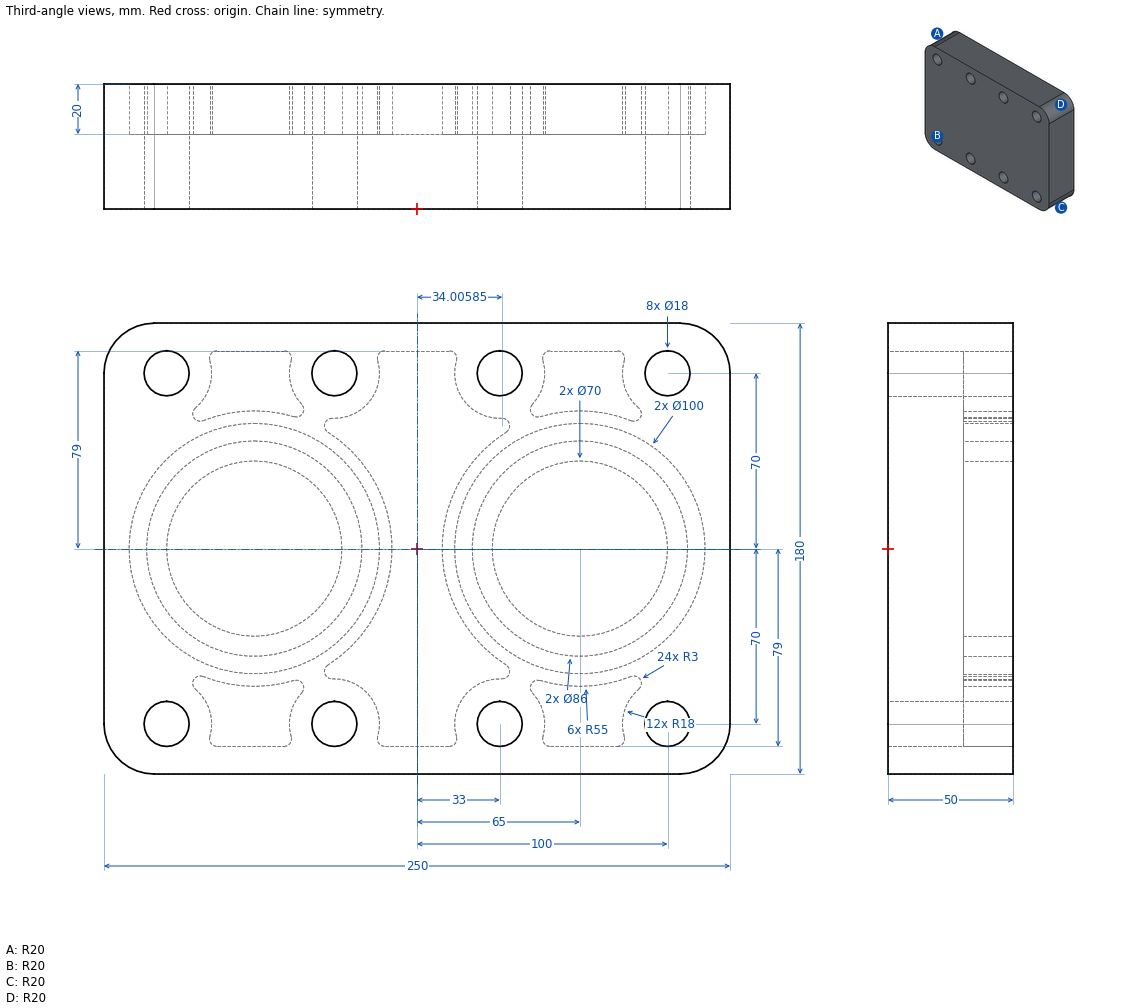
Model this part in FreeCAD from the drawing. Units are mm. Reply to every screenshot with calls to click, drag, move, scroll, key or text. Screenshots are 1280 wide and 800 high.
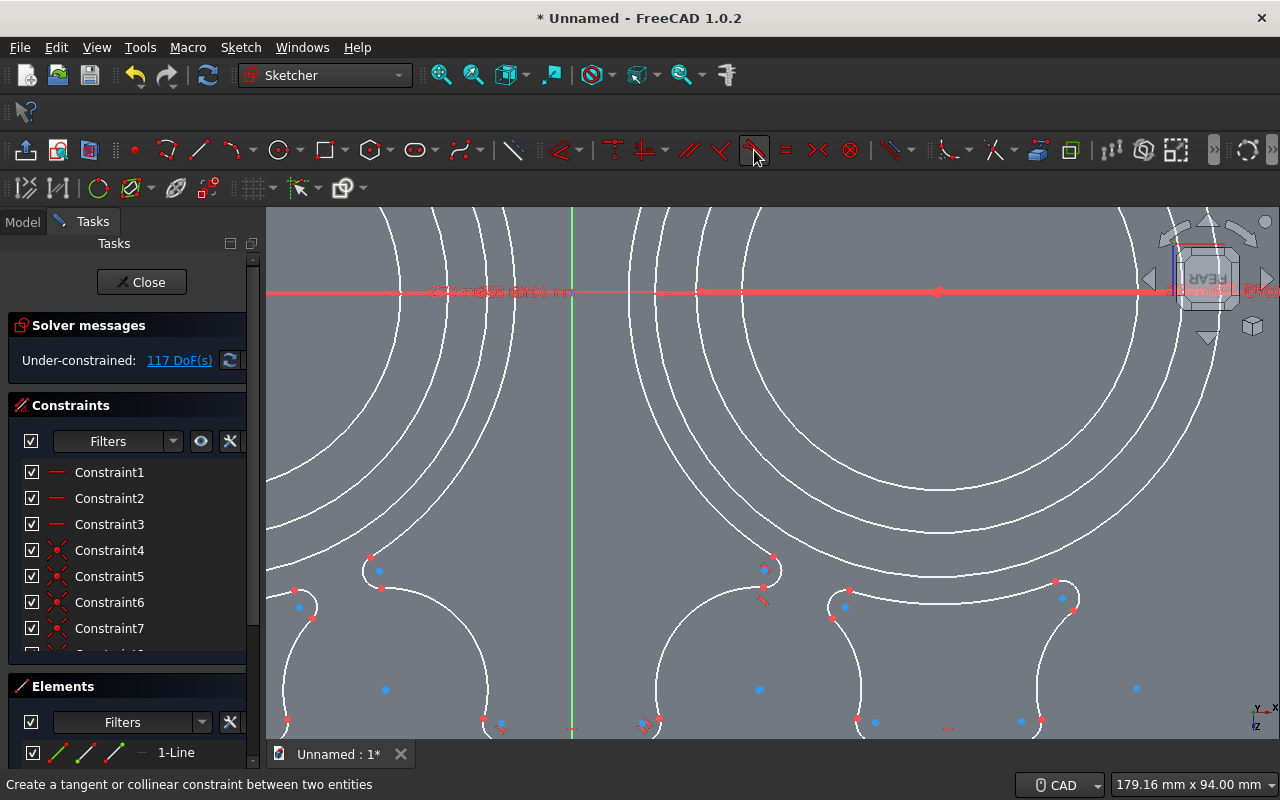
click(654, 416)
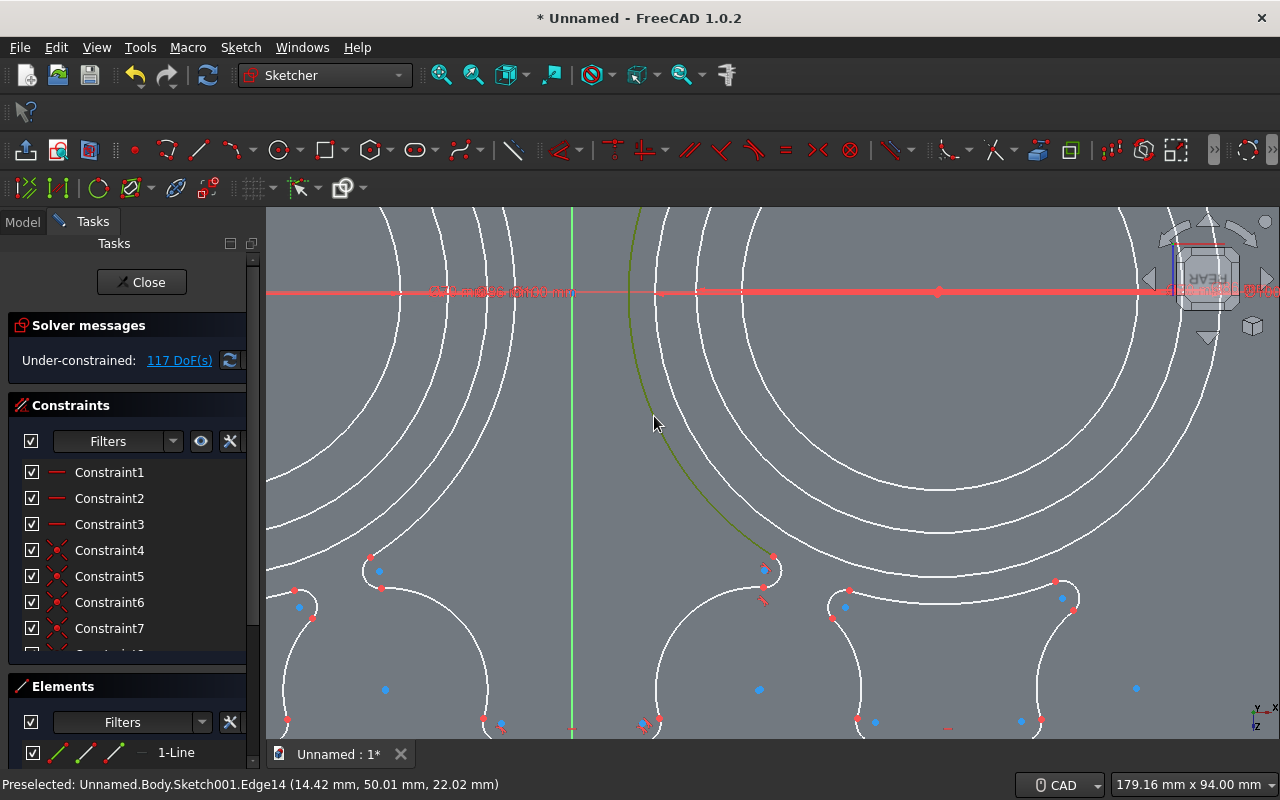
scroll(781, 578, down, 5)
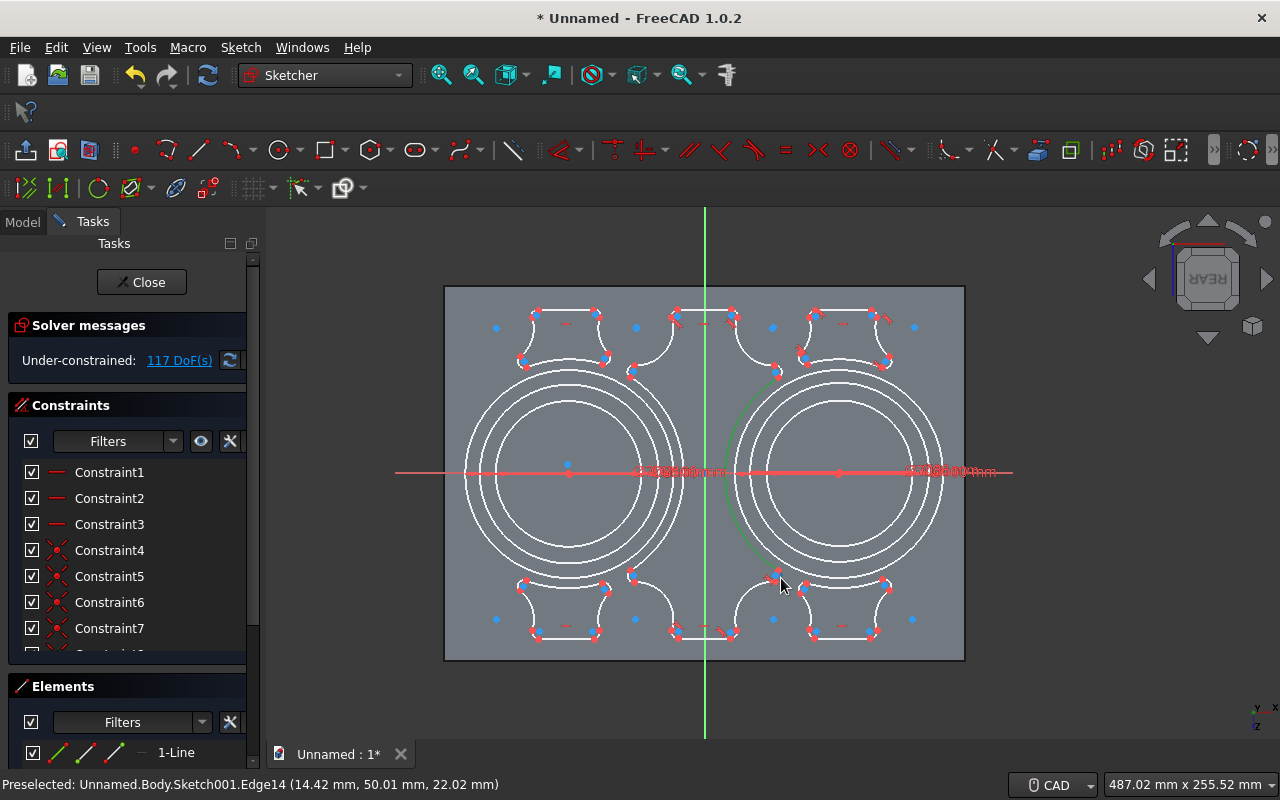
scroll(782, 374, up, 5)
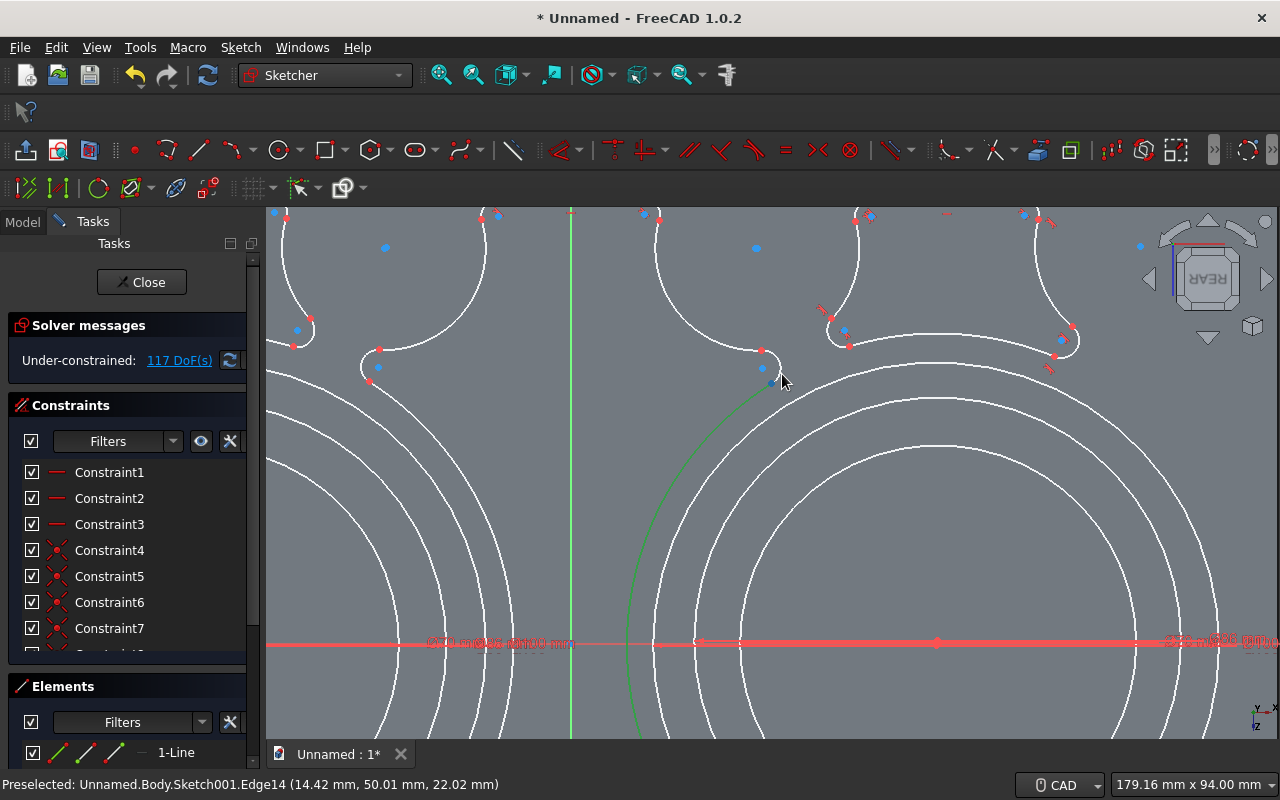
click(780, 373)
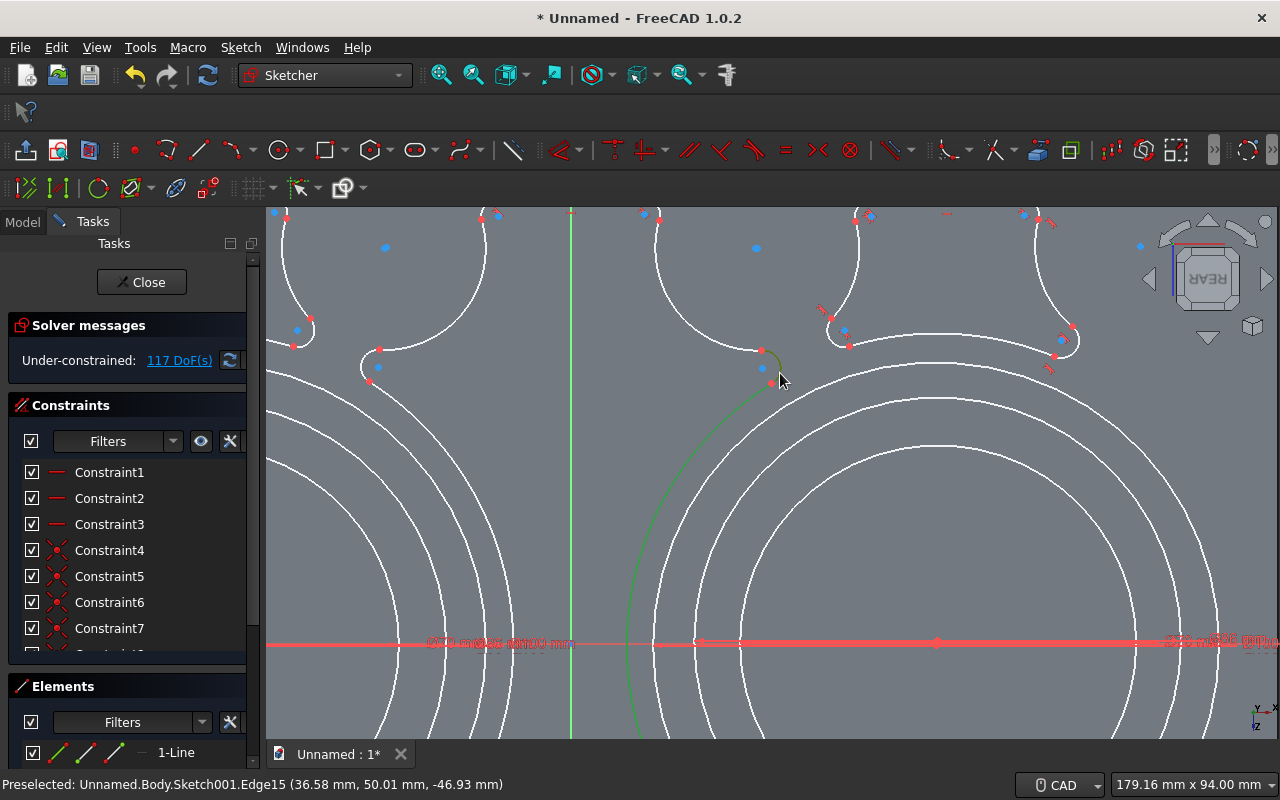
click(754, 150)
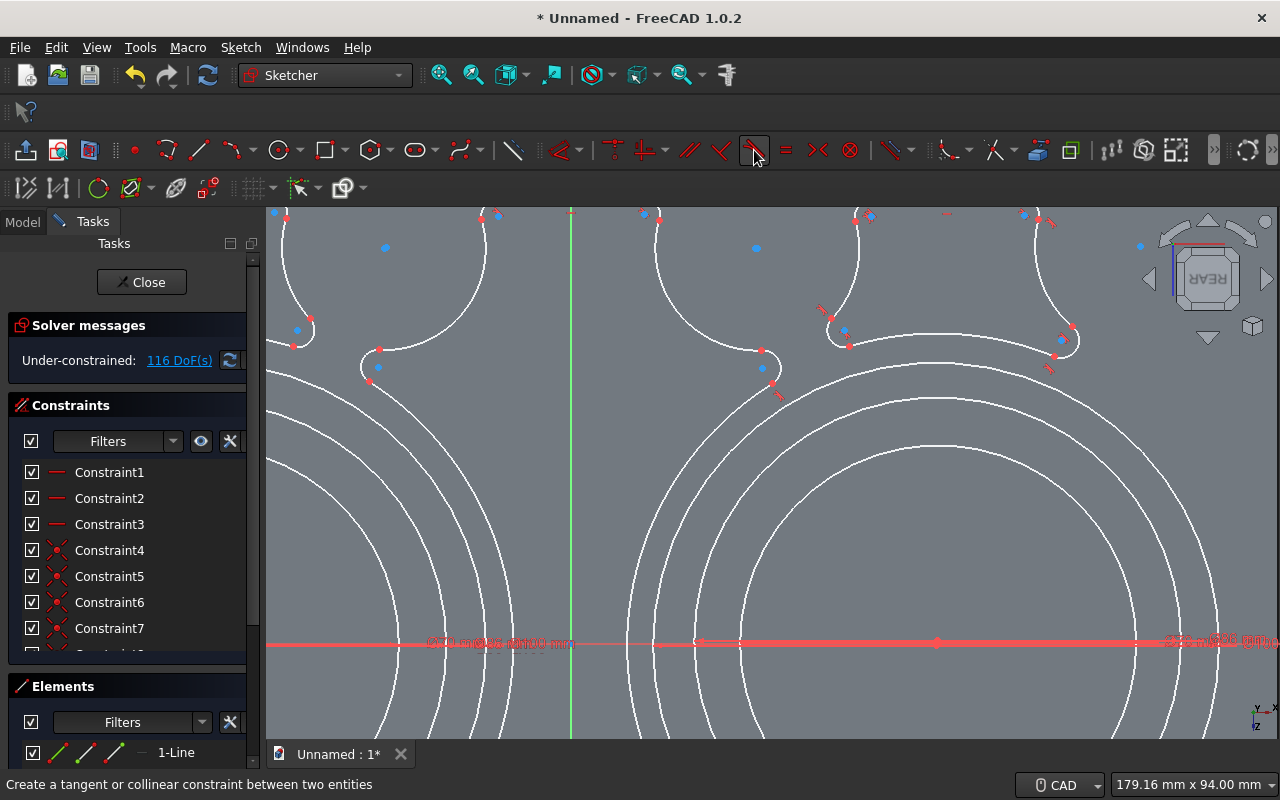
click(780, 372)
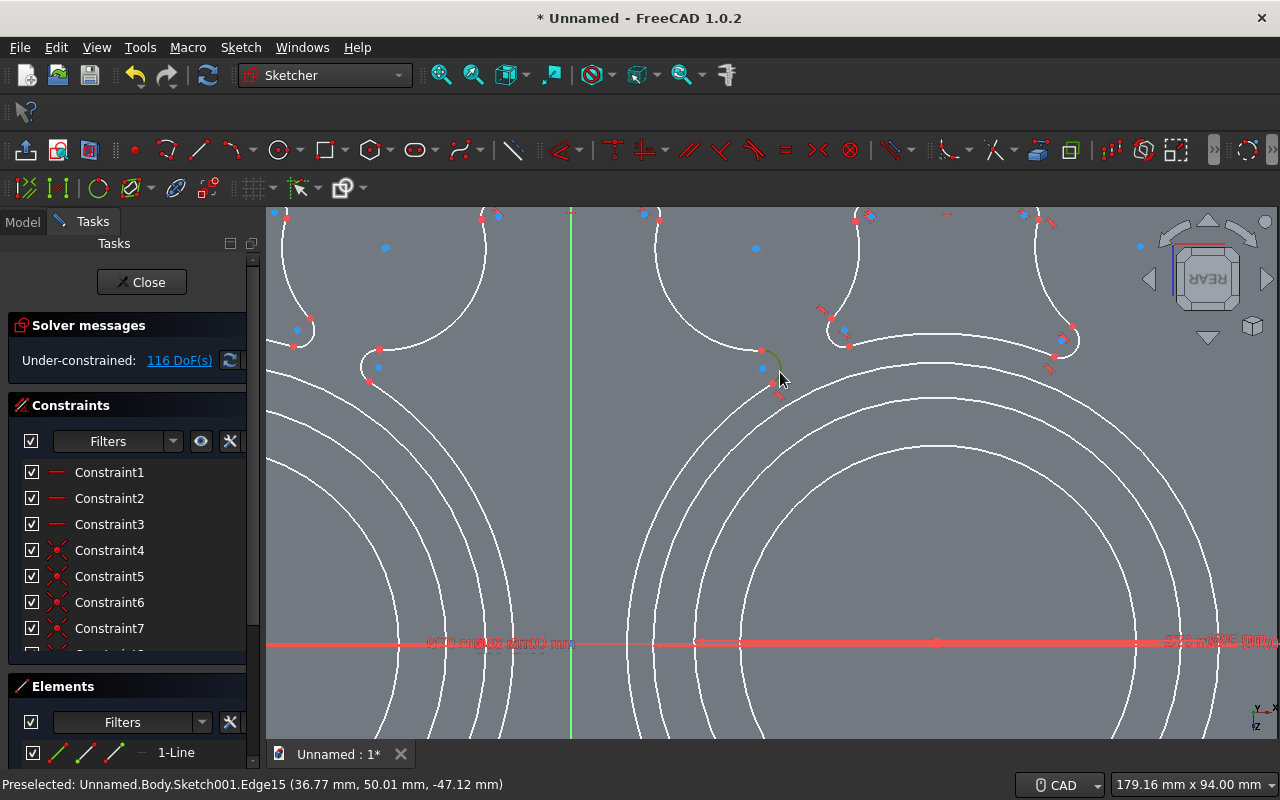
click(660, 278)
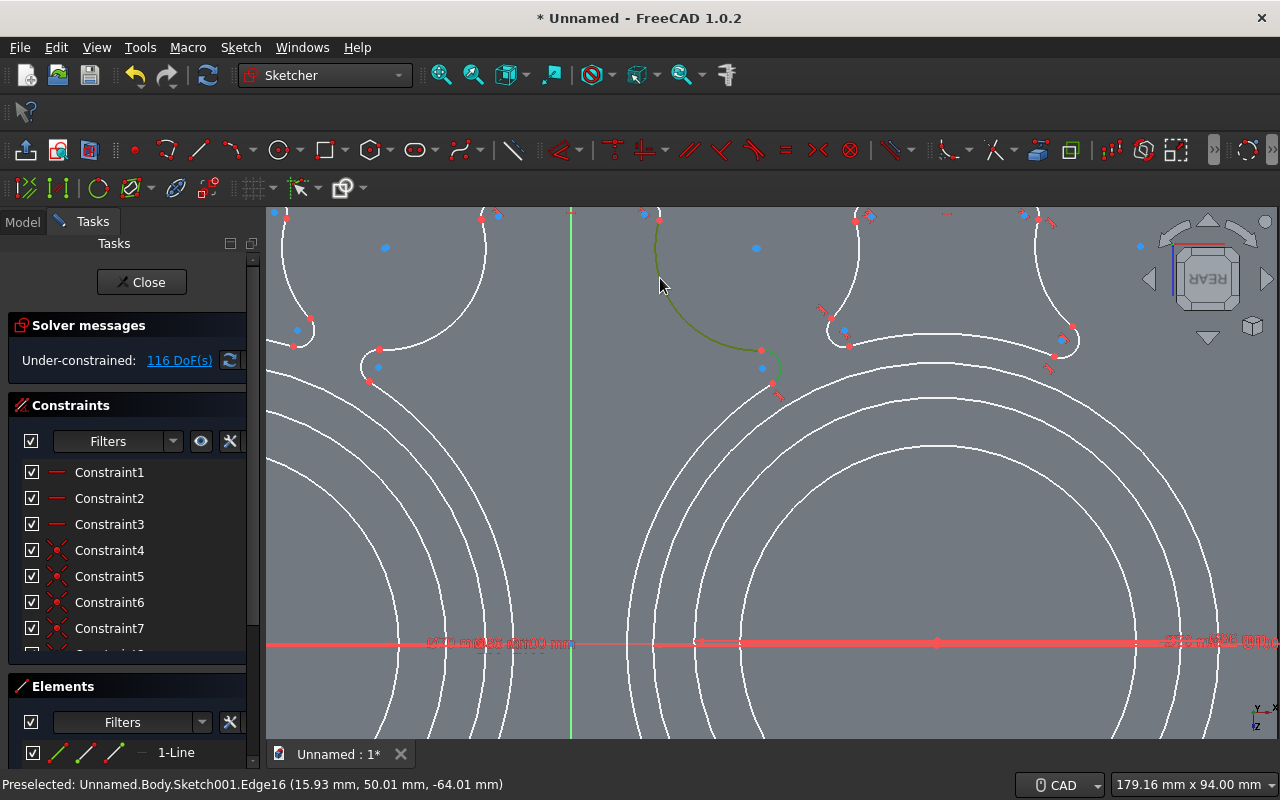
click(754, 150)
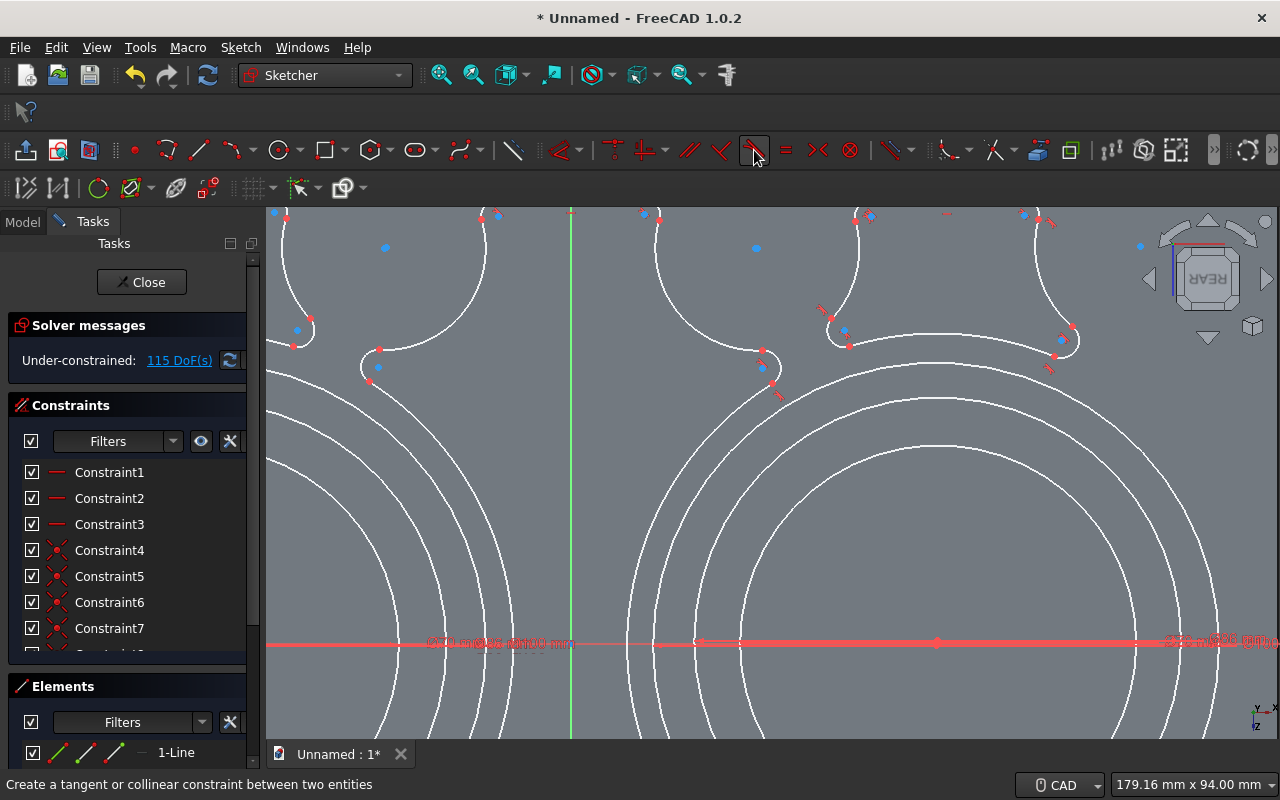
click(660, 278)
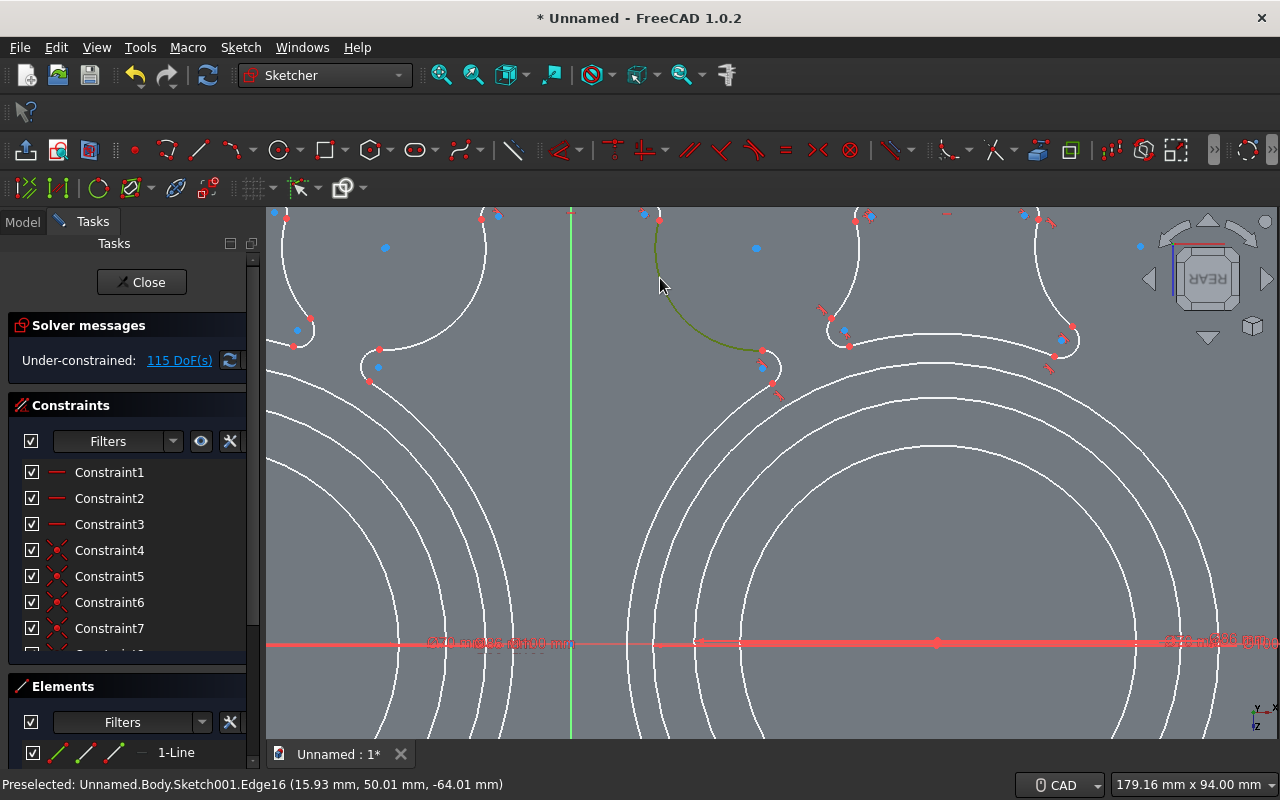
scroll(782, 374, down, 5)